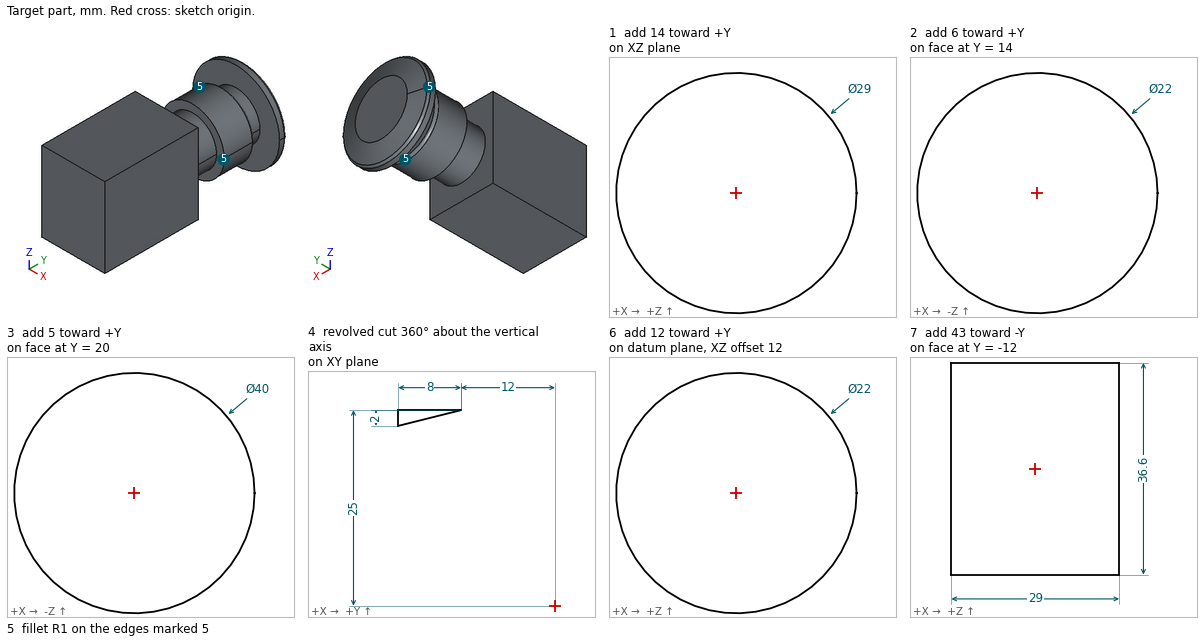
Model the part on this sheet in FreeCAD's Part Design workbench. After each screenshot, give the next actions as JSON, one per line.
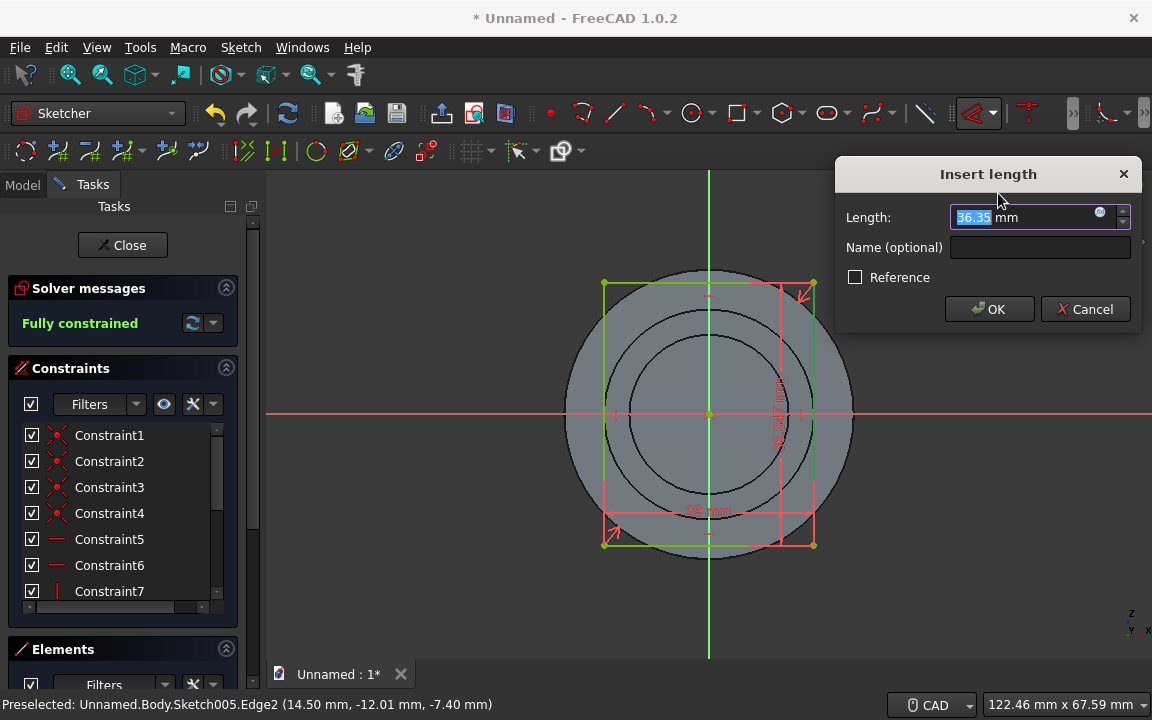
{"action": "type", "text": "36.6"}
{"action": "key", "text": "Return"}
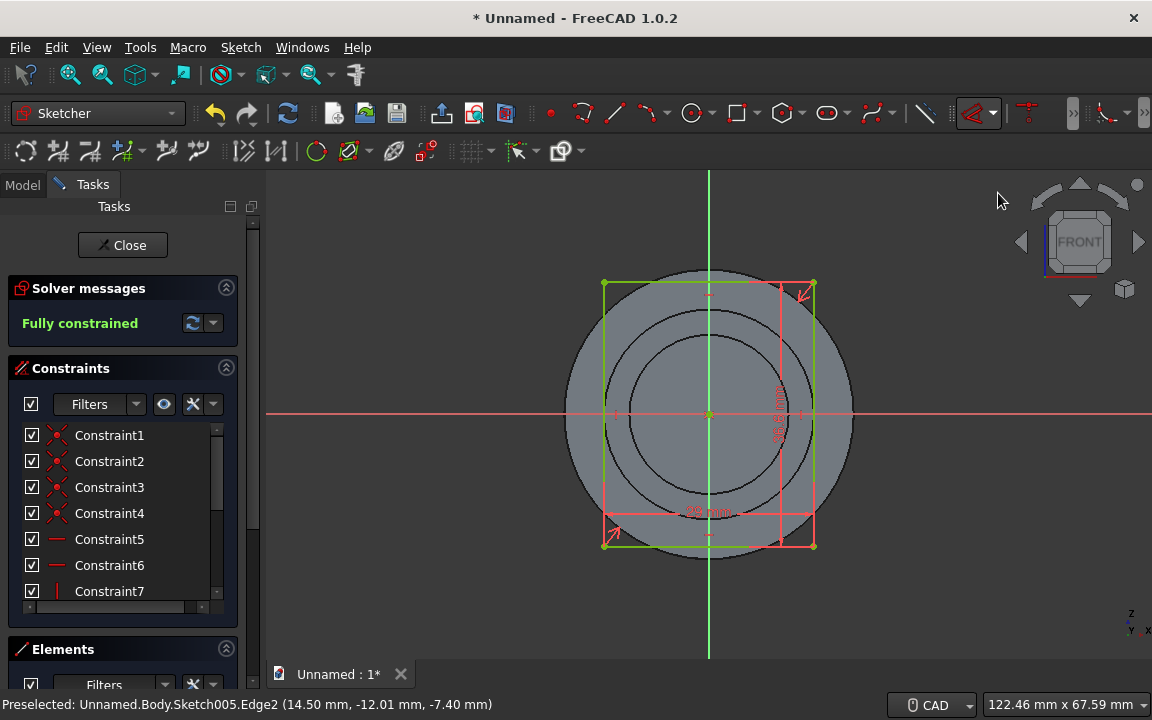
{"action": "left_click", "coordinate": [123, 245]}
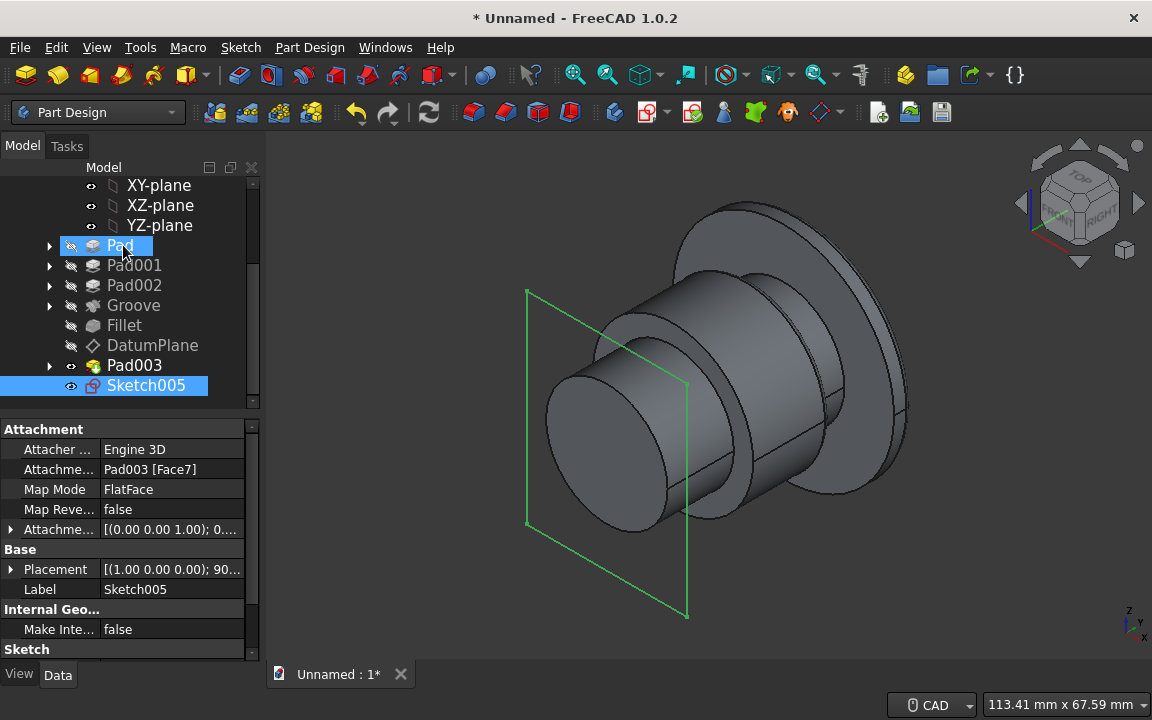
{"action": "left_click", "coordinate": [26, 76]}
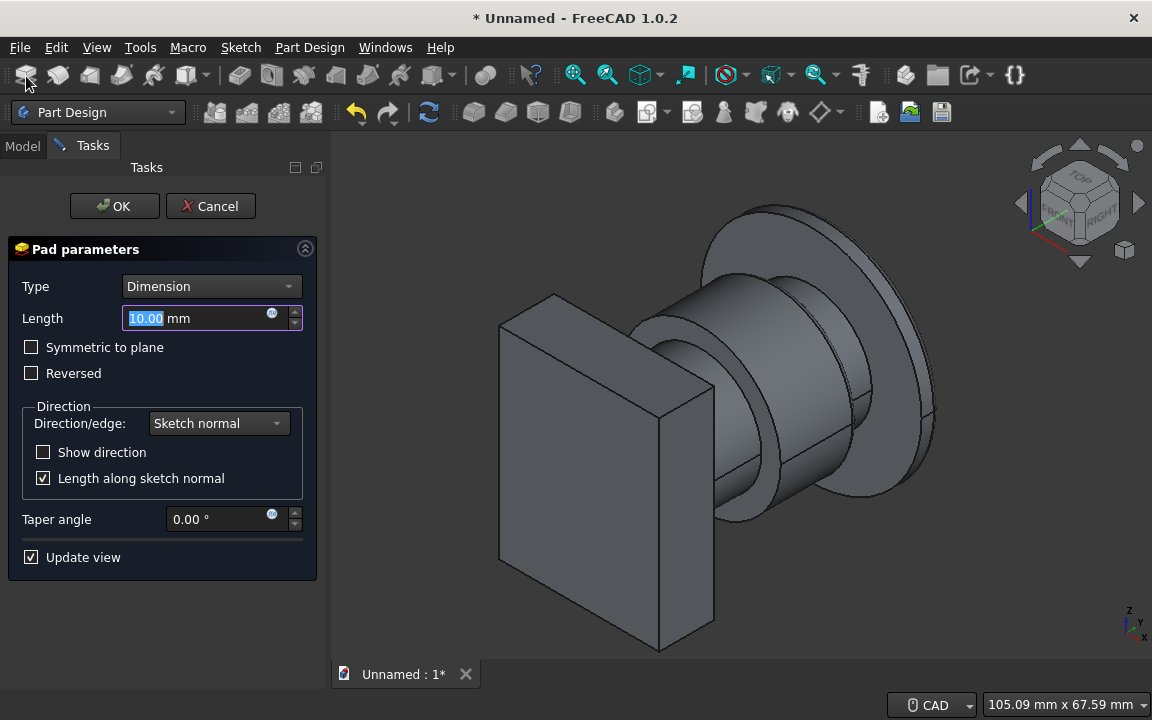
{"action": "type", "text": "43"}
{"action": "key", "text": "Tab"}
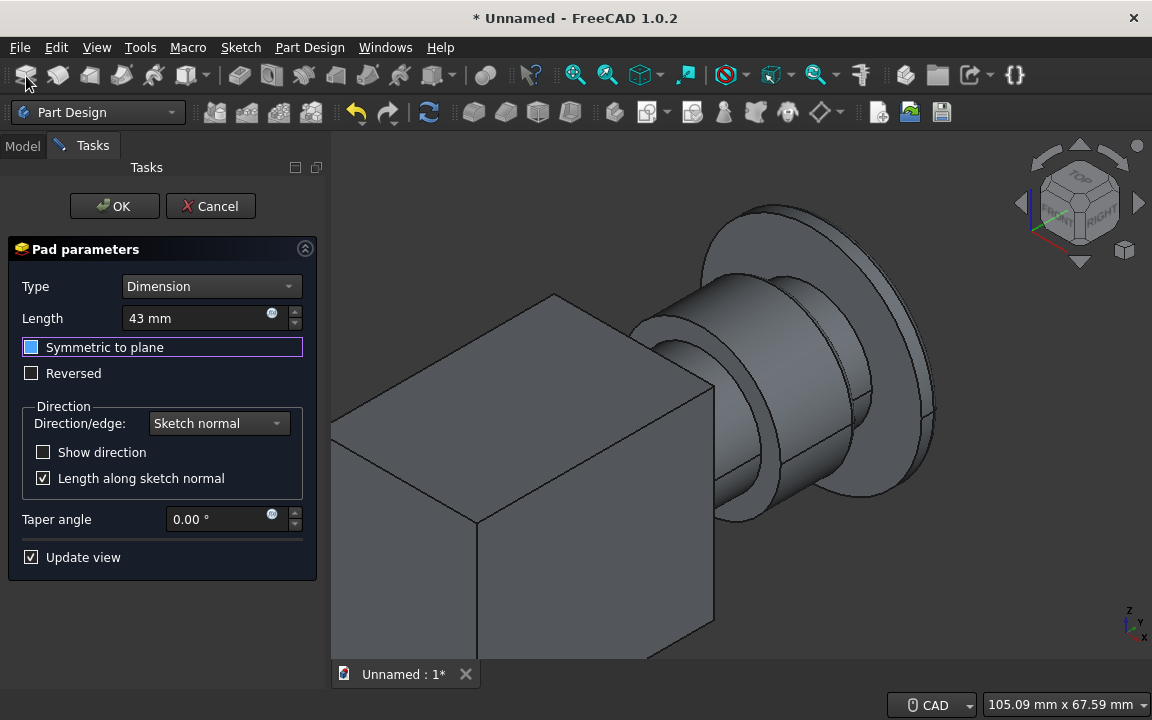
{"action": "left_click", "coordinate": [115, 206]}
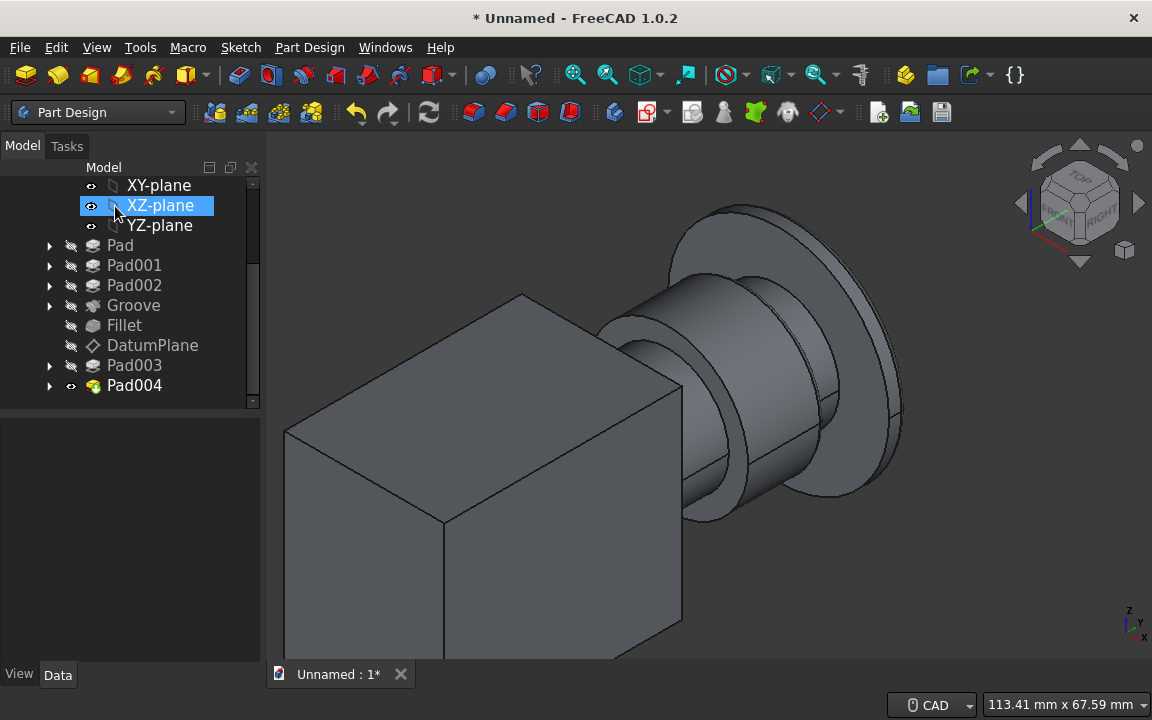
{"action": "key", "text": "v f"}